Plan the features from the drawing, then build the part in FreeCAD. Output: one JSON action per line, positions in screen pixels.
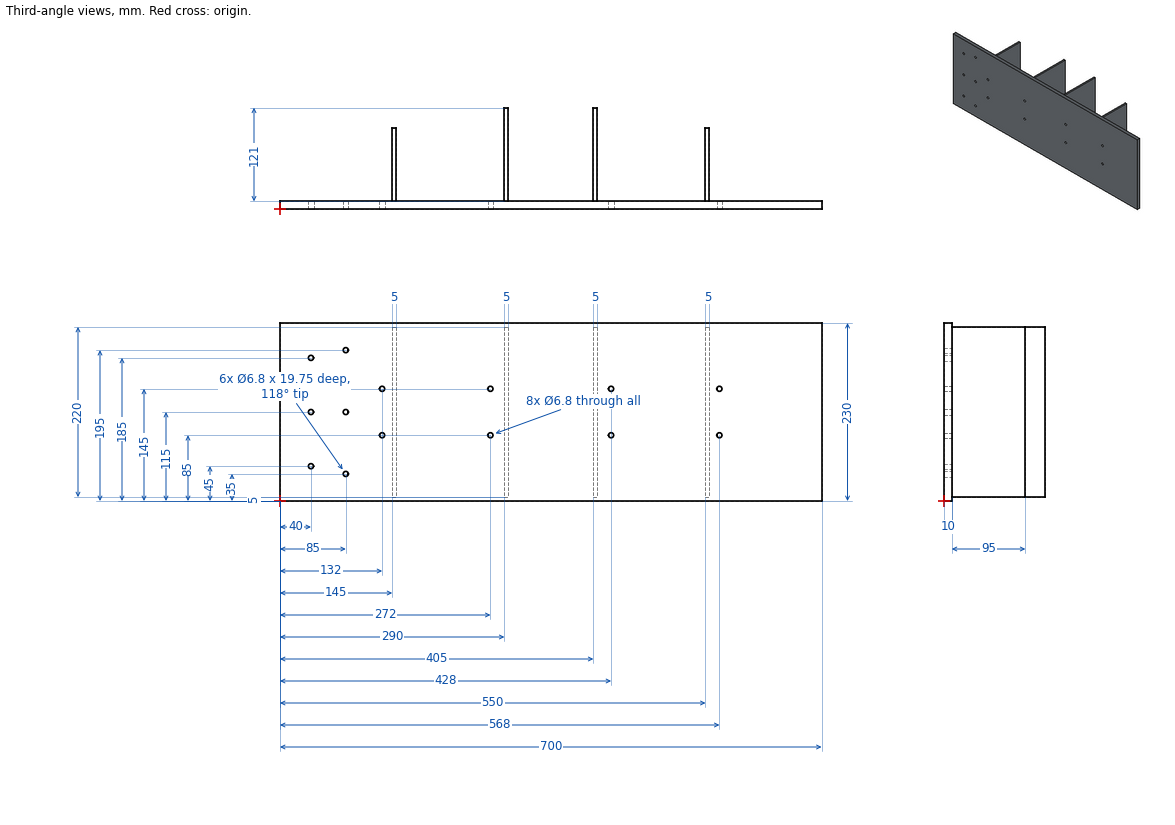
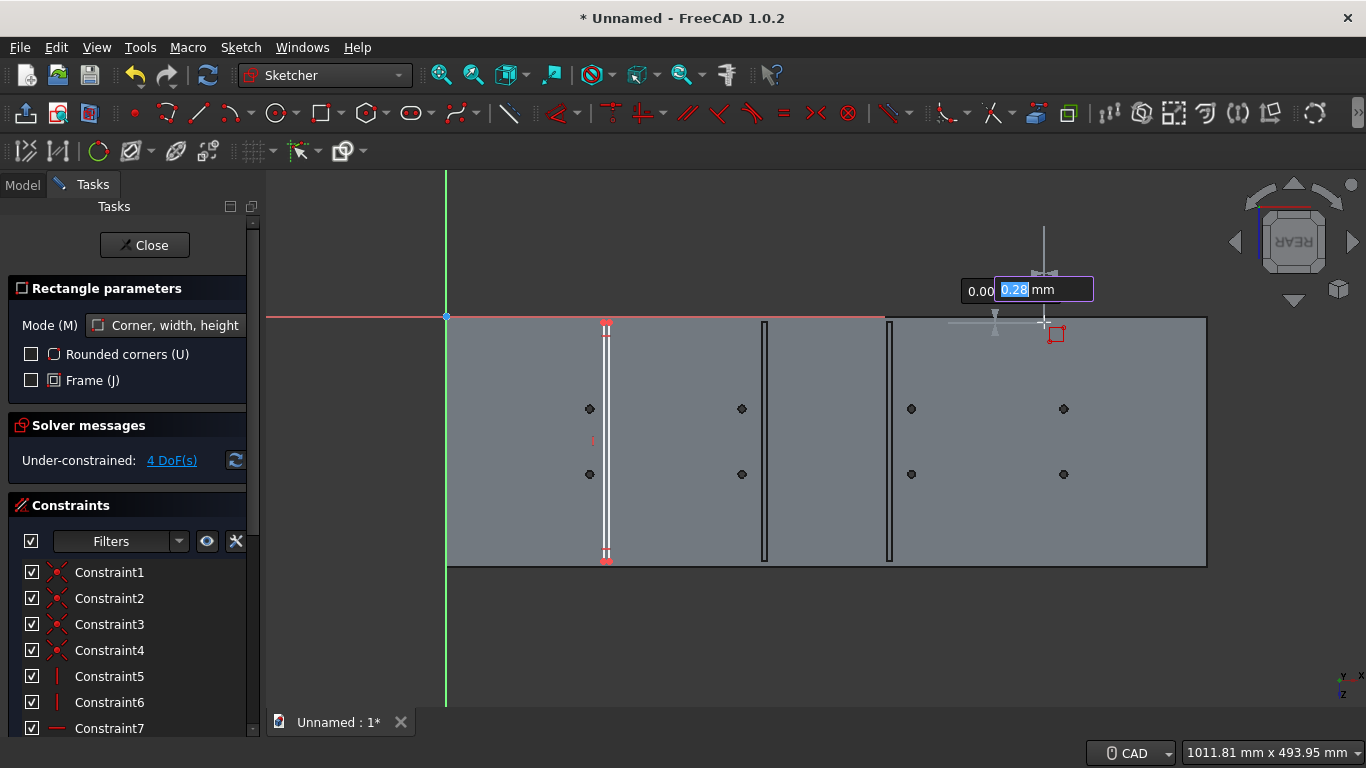
{"action": "left_click", "coordinate": [1050, 561]}
{"action": "key", "text": "Escape"}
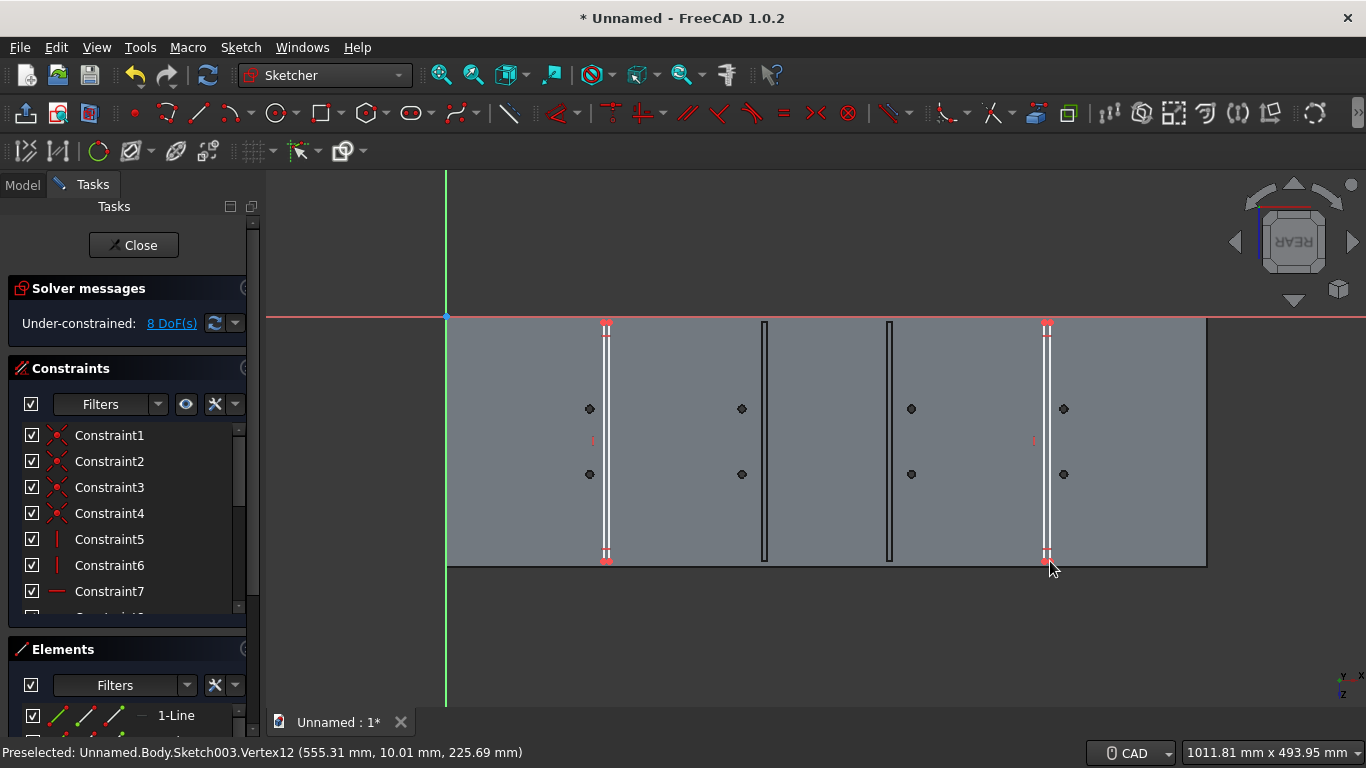
{"action": "left_click", "coordinate": [556, 114]}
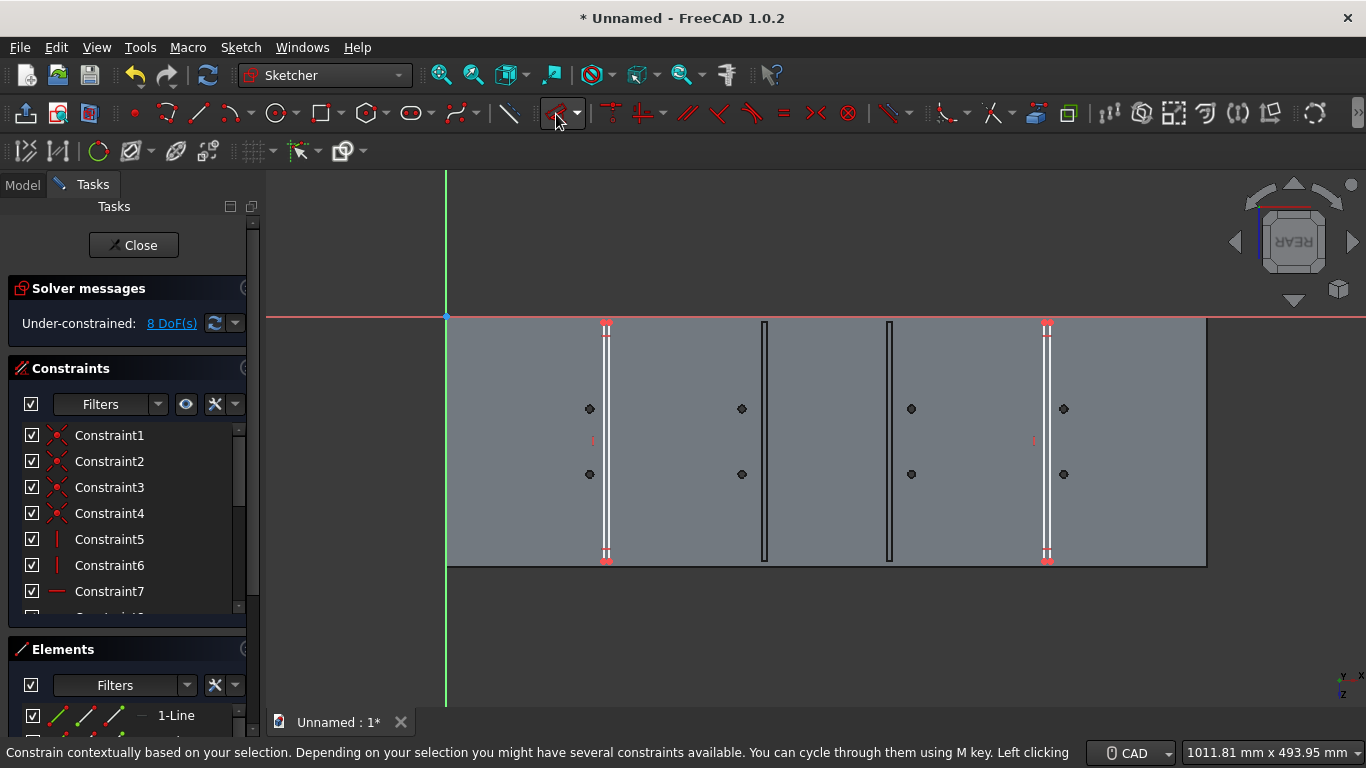
{"action": "scroll", "coordinate": [606, 562], "scroll_direction": "up", "scroll_amount": 10}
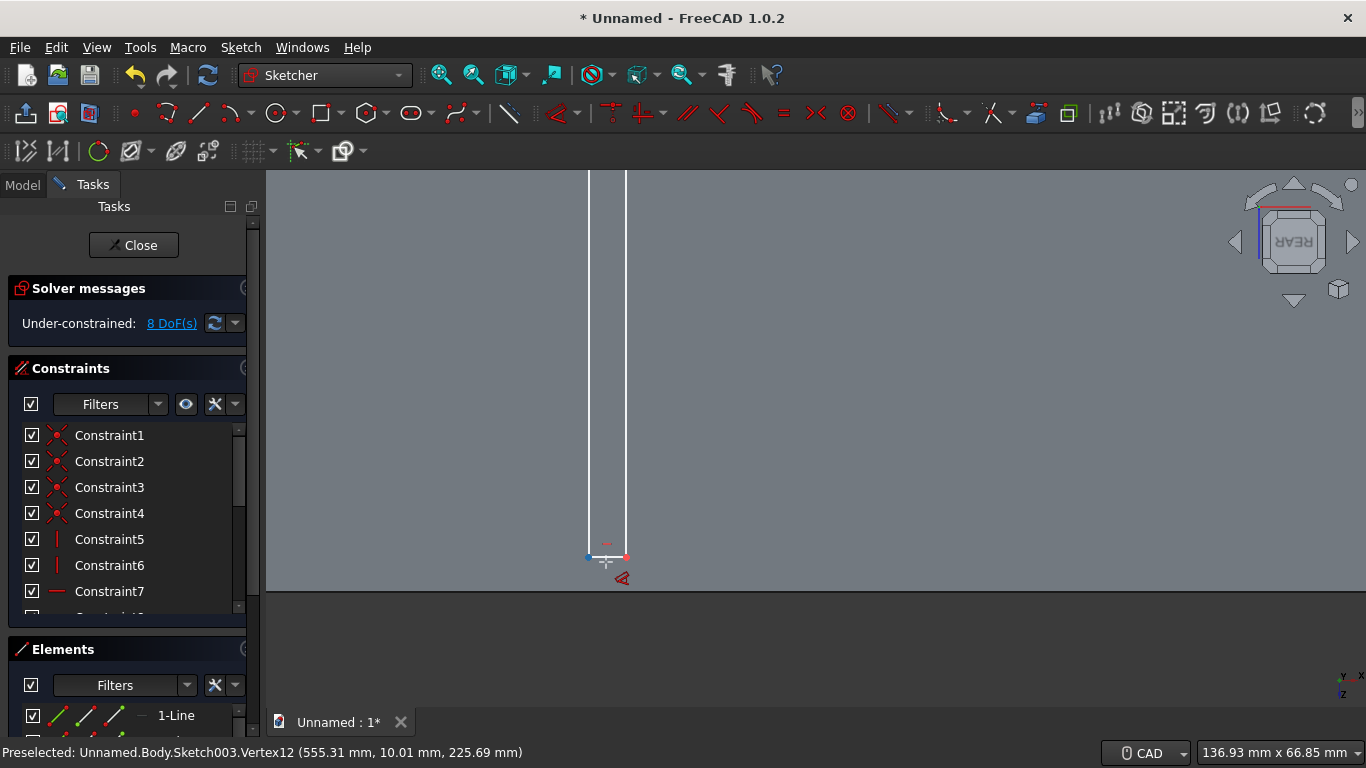
{"action": "left_click", "coordinate": [607, 557]}
{"action": "left_click", "coordinate": [607, 591]}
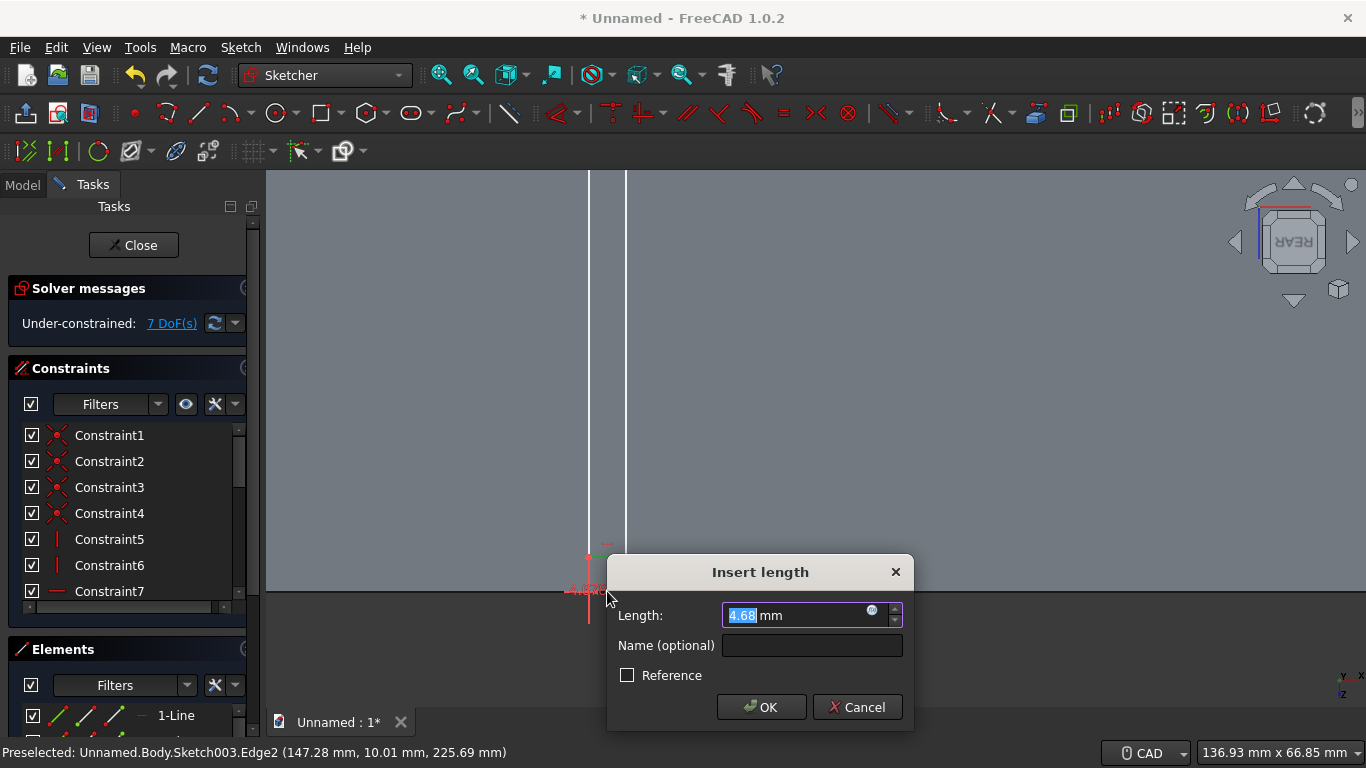
{"action": "type", "text": "5"}
{"action": "key", "text": "Return"}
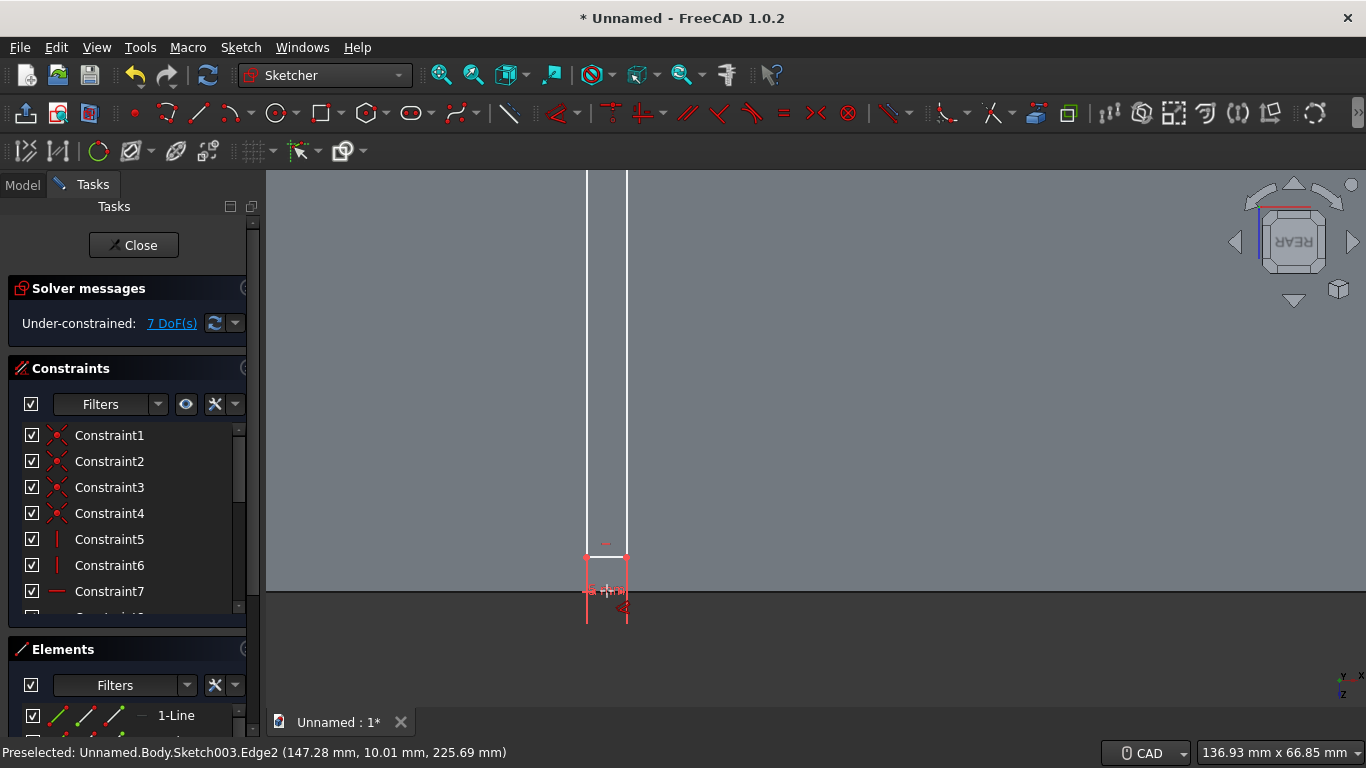
{"action": "scroll", "coordinate": [606, 562], "scroll_direction": "down", "scroll_amount": 10}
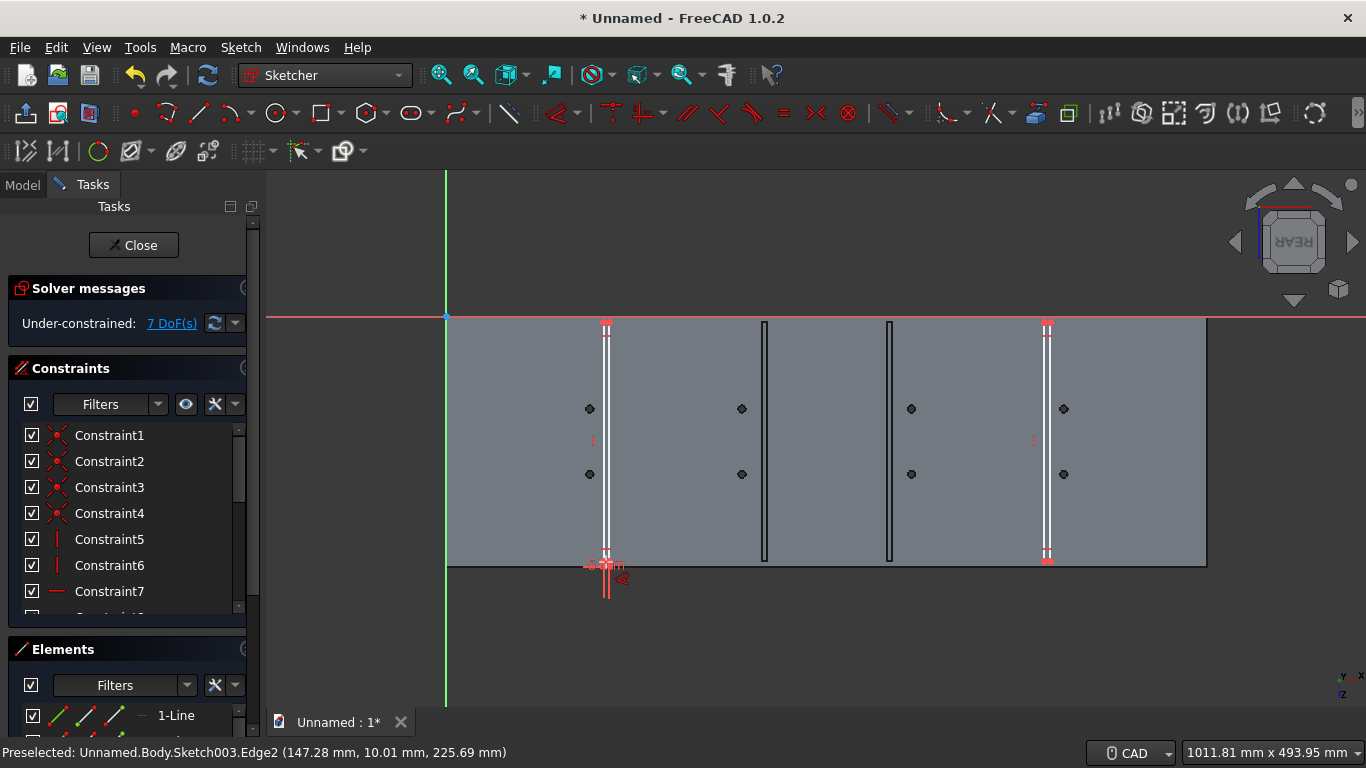
{"action": "scroll", "coordinate": [1046, 562], "scroll_direction": "up", "scroll_amount": 11}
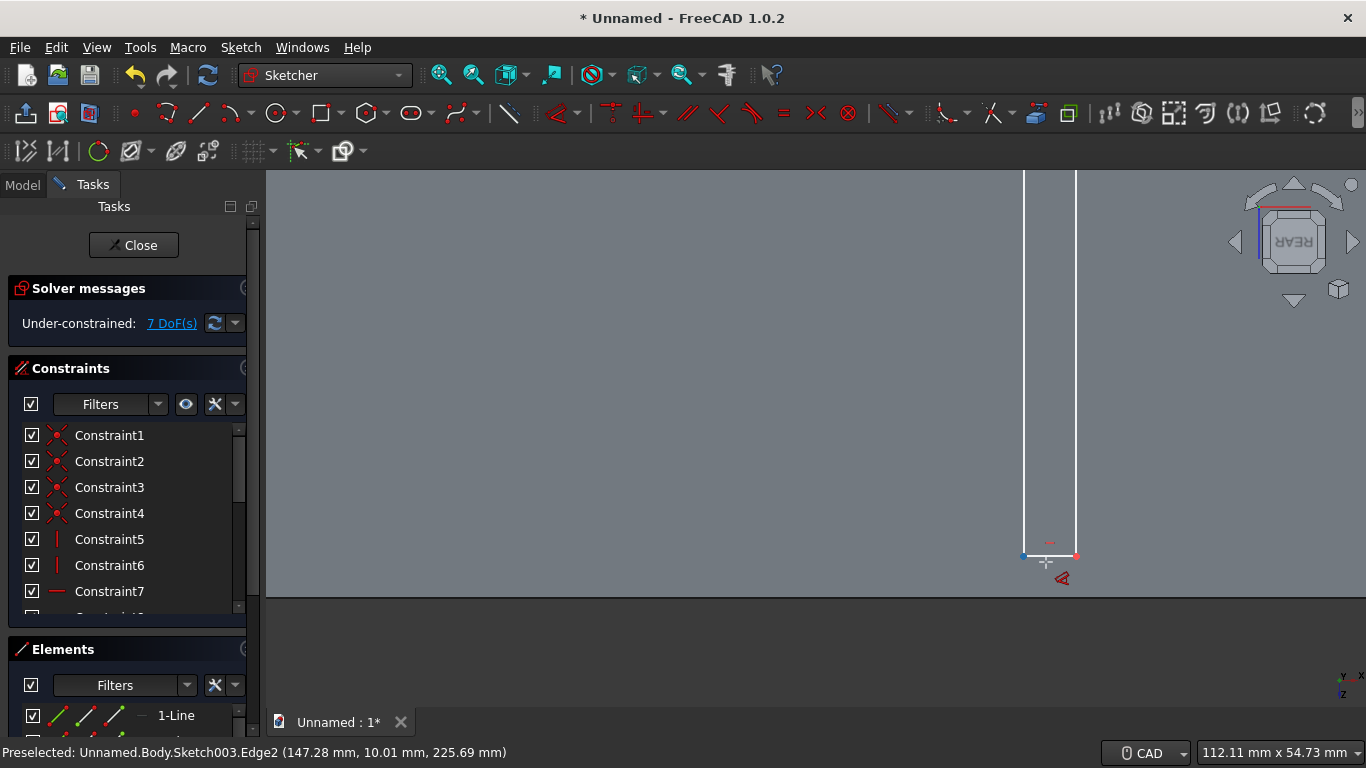
{"action": "left_click", "coordinate": [1040, 556]}
{"action": "left_click", "coordinate": [1050, 590]}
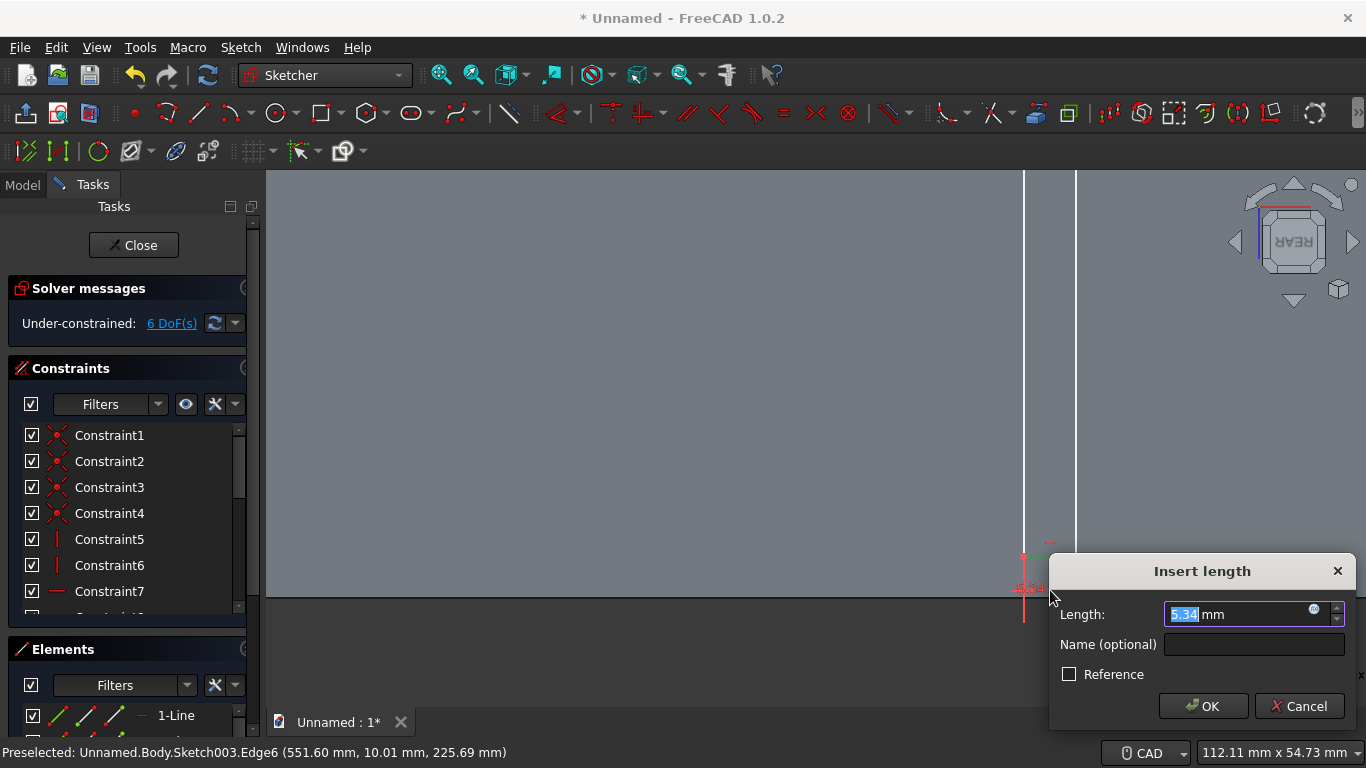
{"action": "type", "text": "5"}
{"action": "key", "text": "Return"}